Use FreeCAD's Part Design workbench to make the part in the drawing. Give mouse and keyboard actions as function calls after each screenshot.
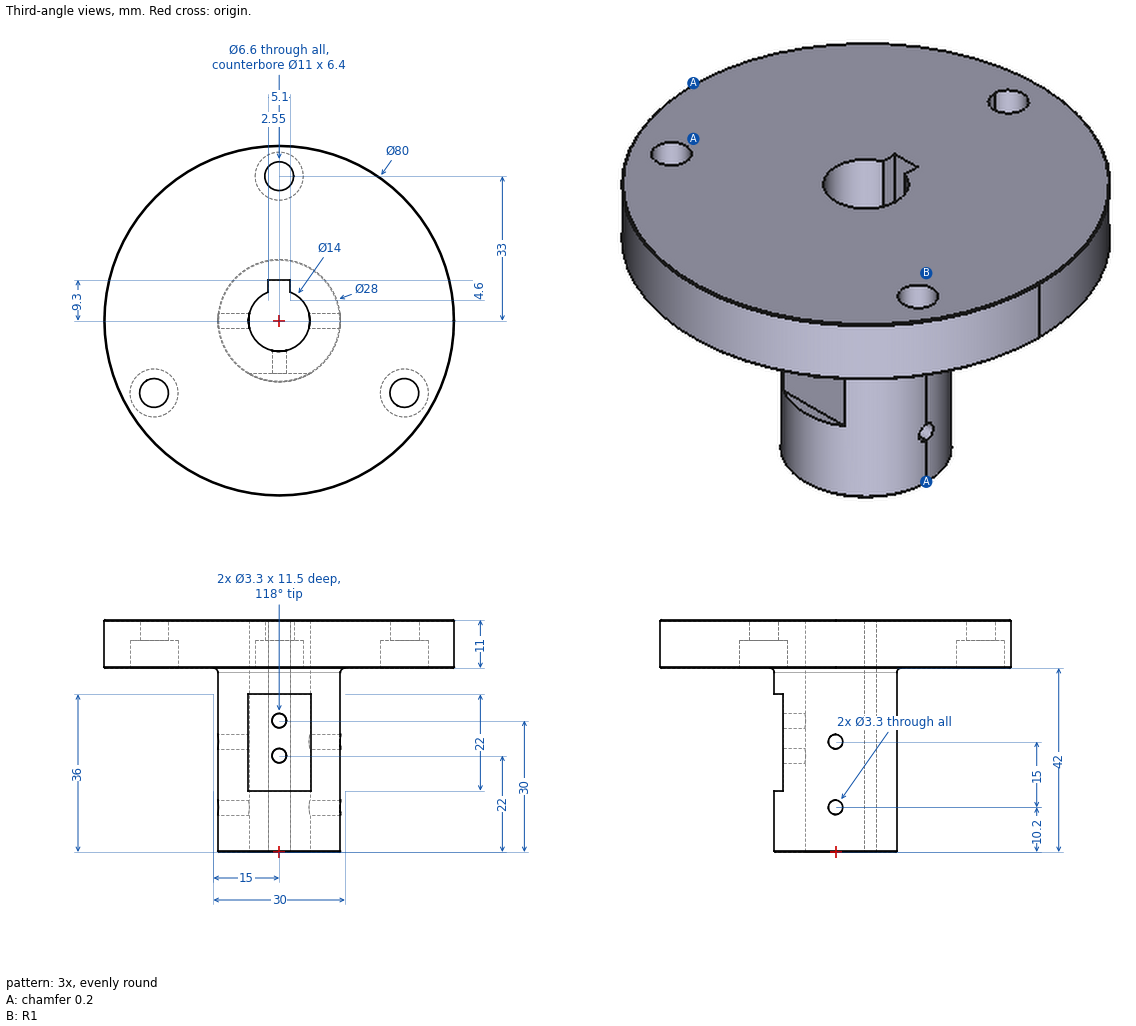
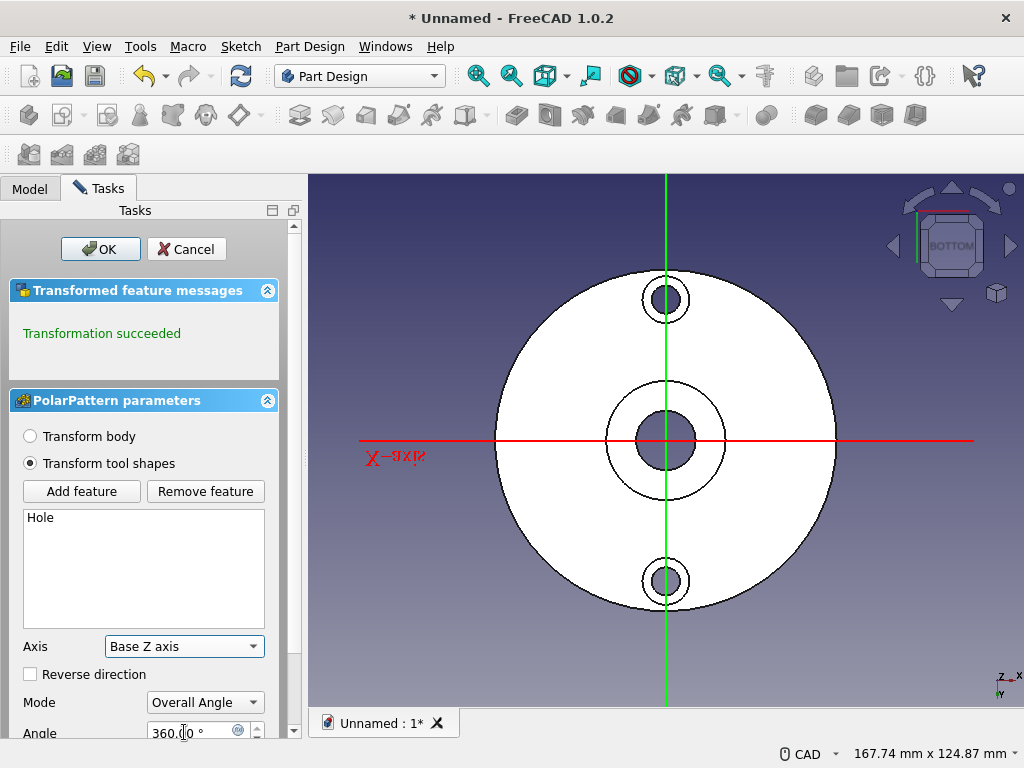
scroll(294, 479, down, 2)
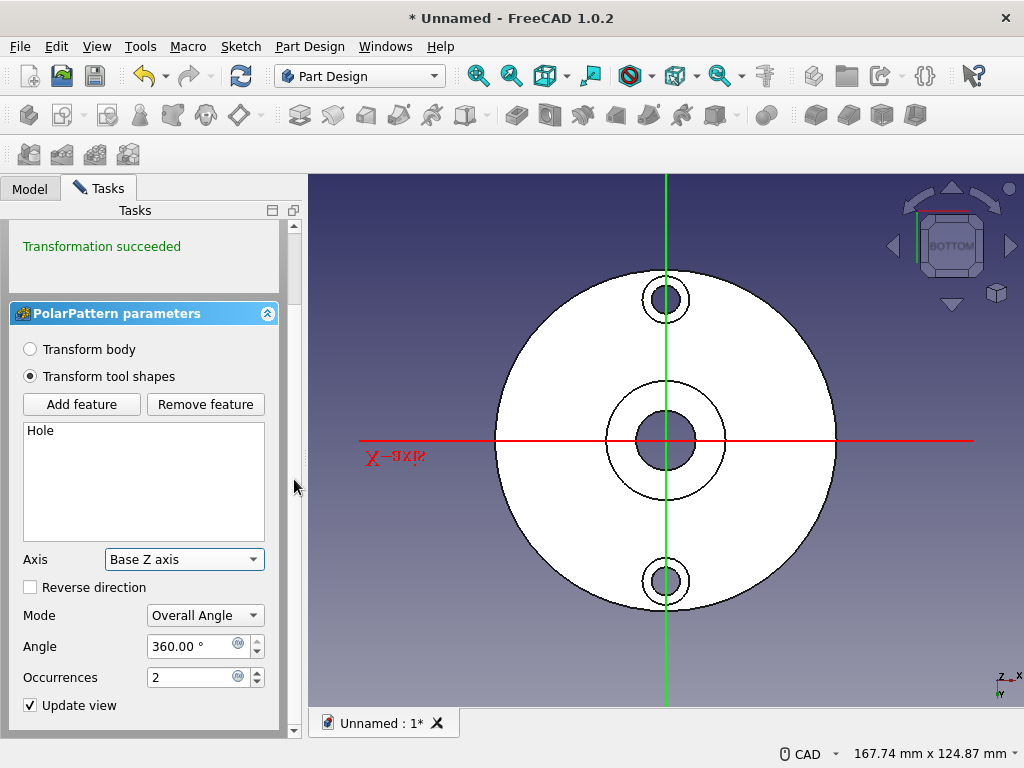
triple_click(199, 678)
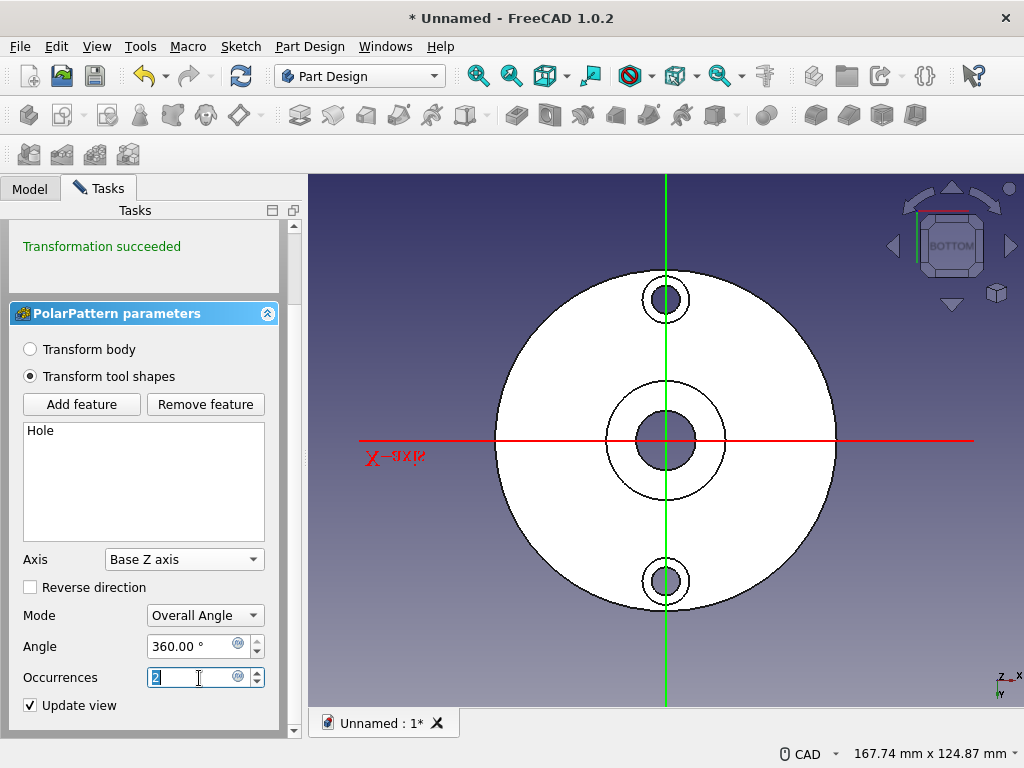
text(3)
key(Tab)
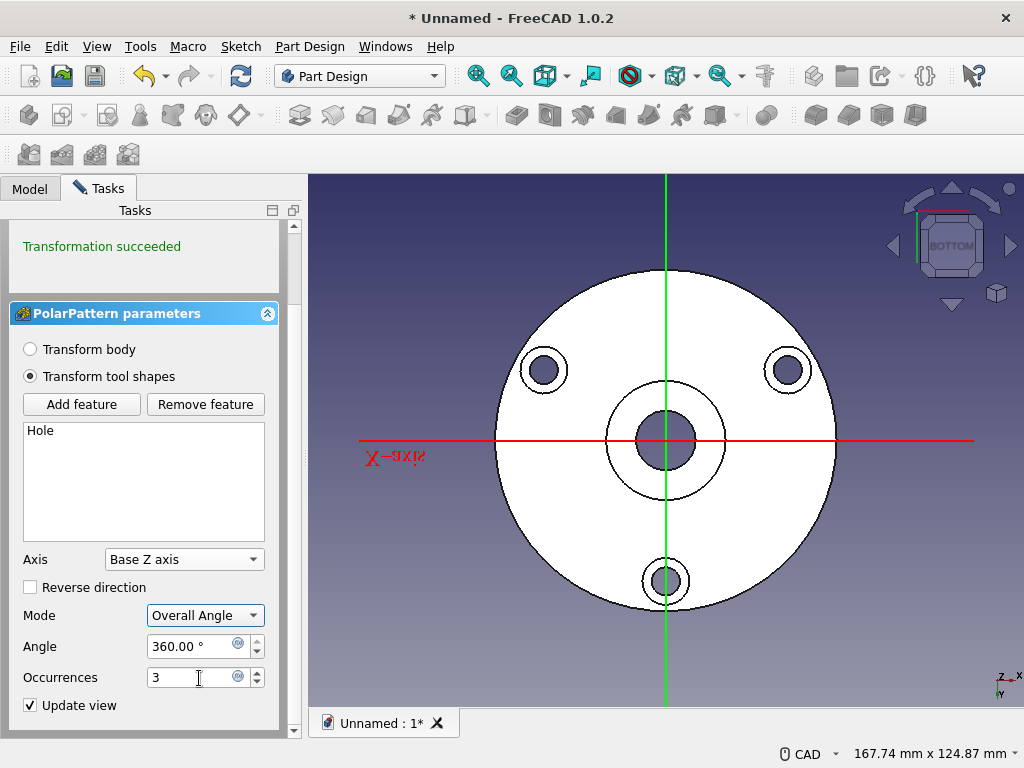
scroll(294, 479, up, 3)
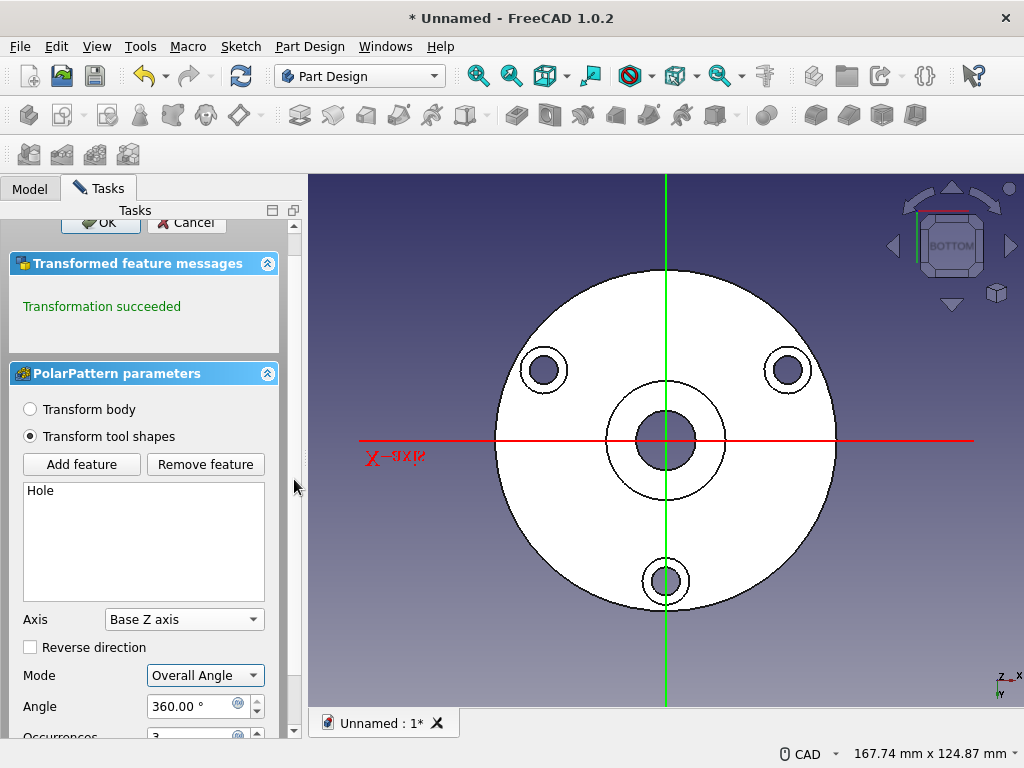
click(101, 249)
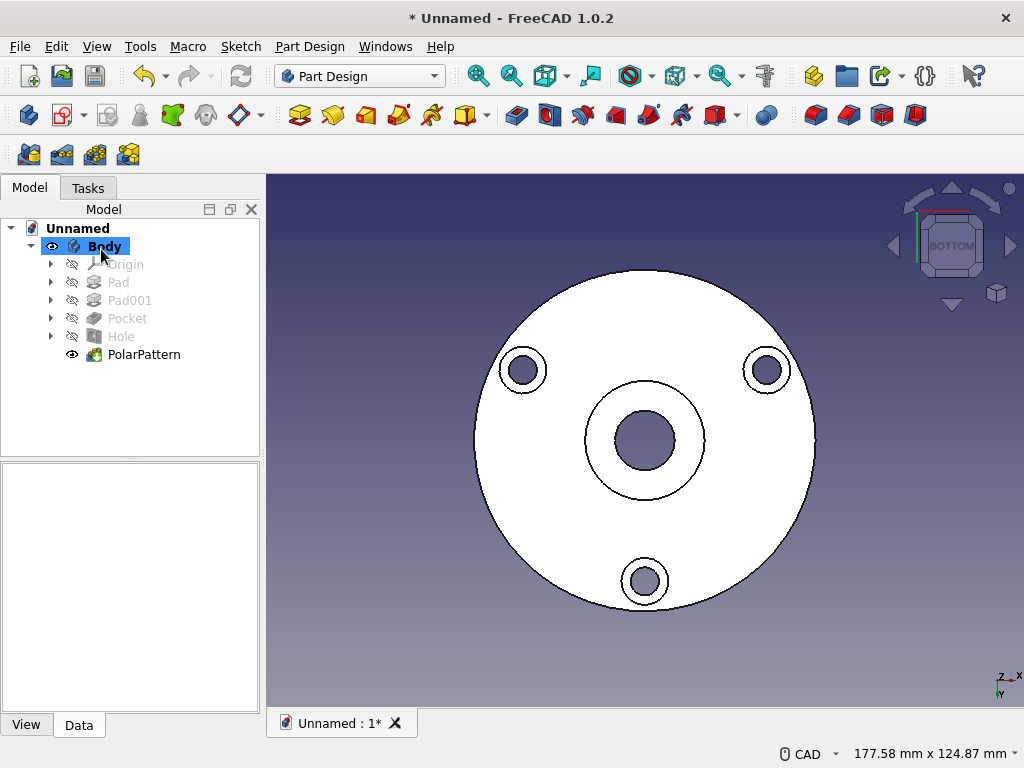
click(51, 264)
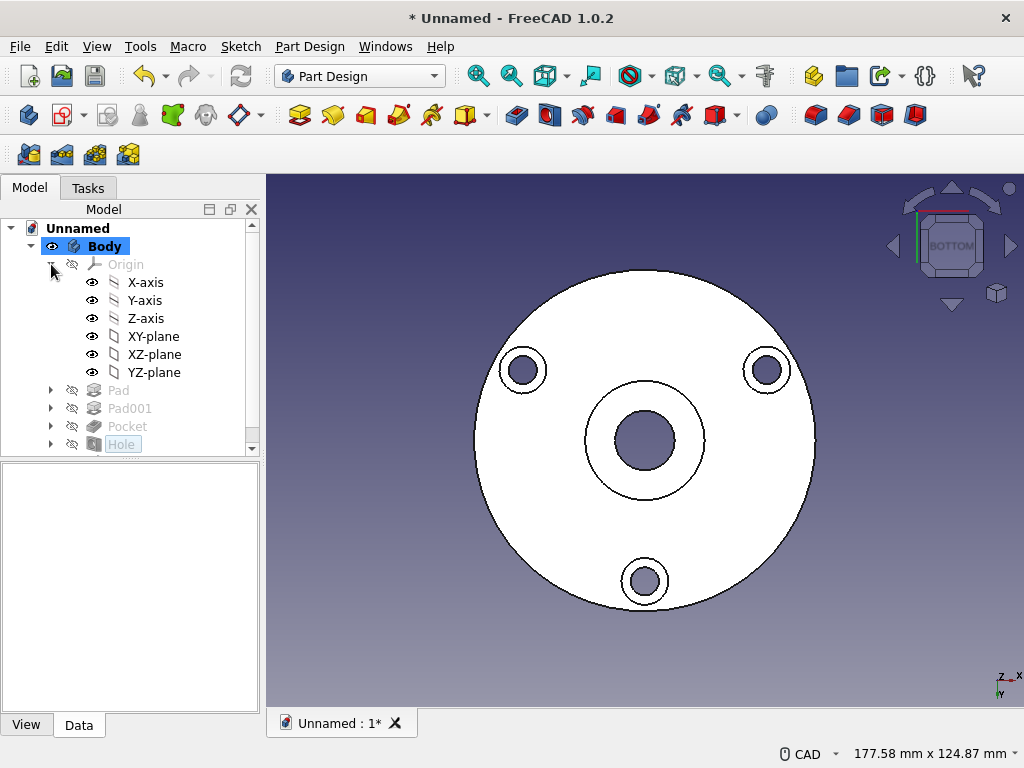
click(137, 354)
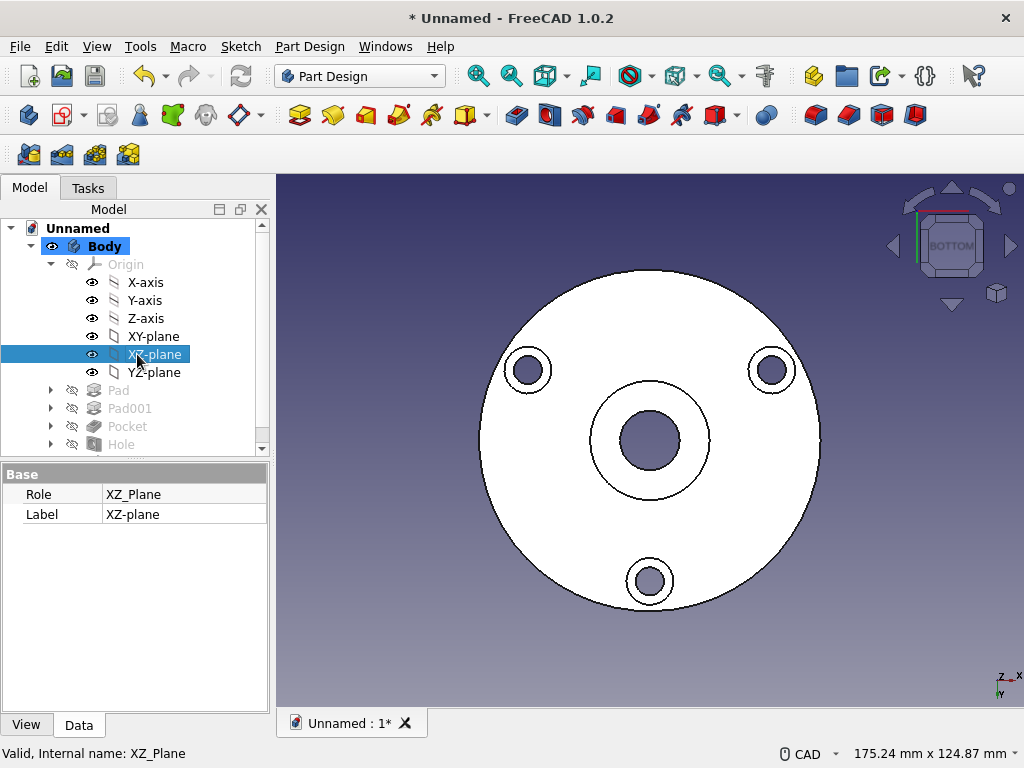
click(238, 116)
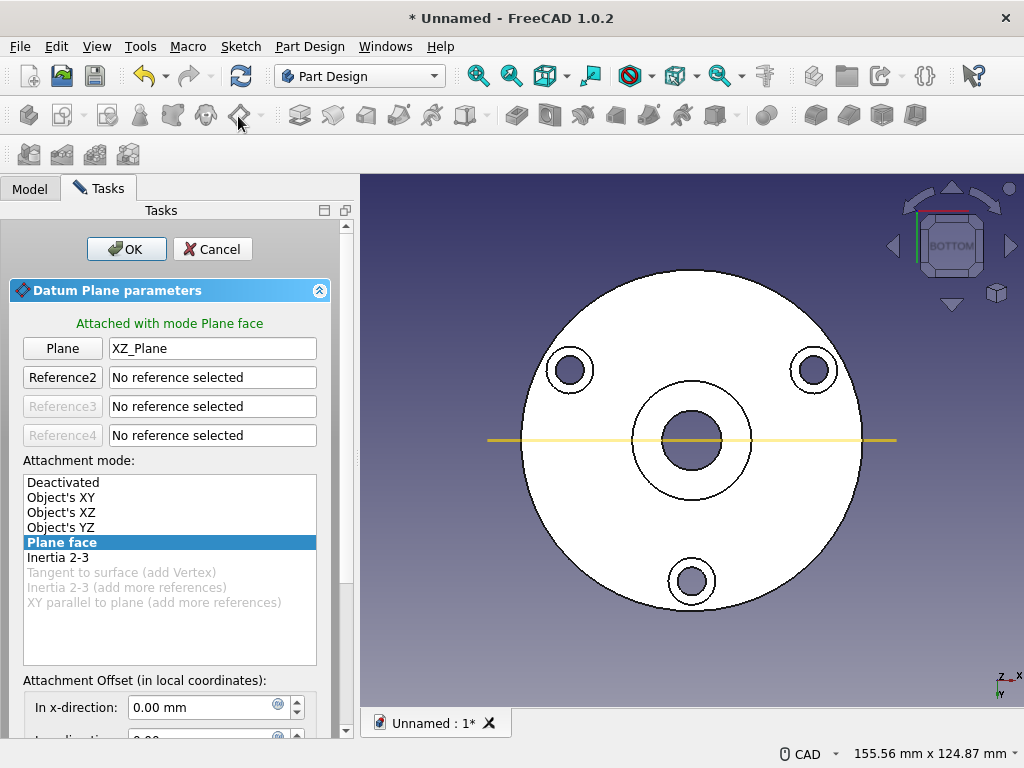
scroll(346, 479, down, 2)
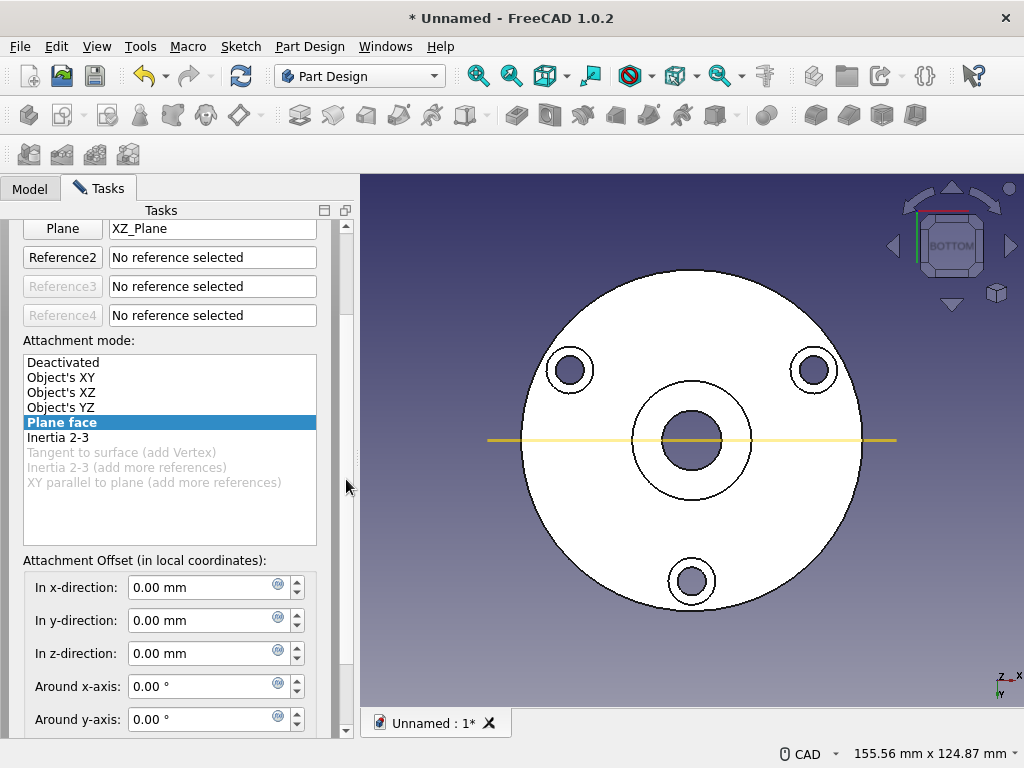
triple_click(210, 654)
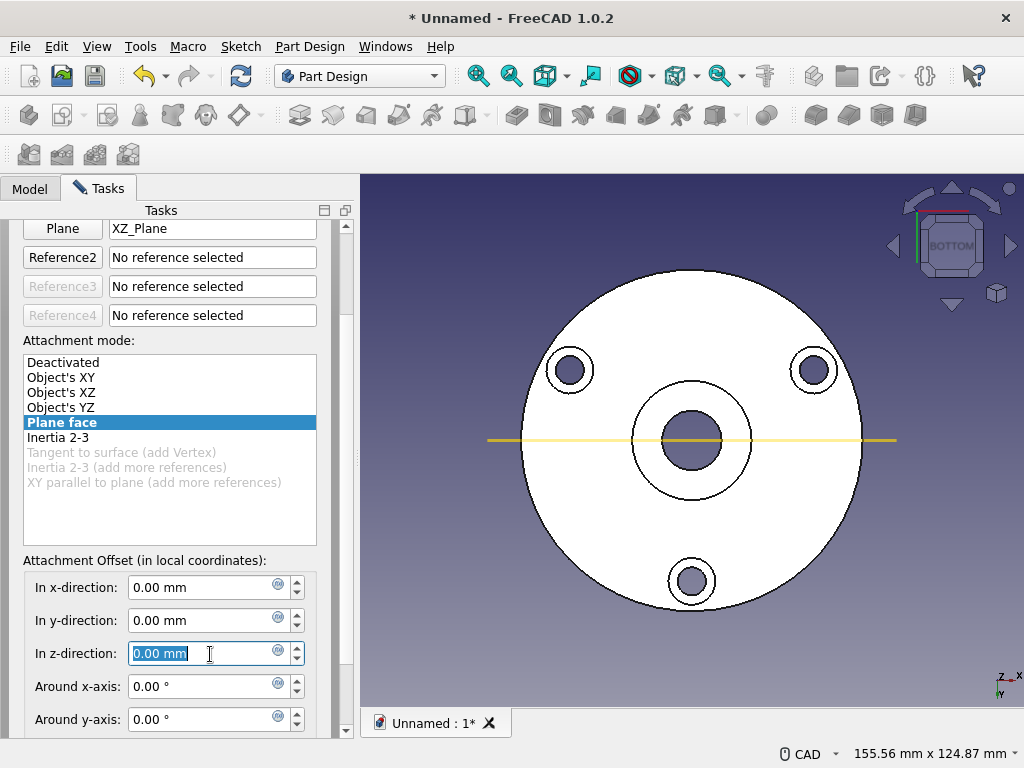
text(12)
key(Tab)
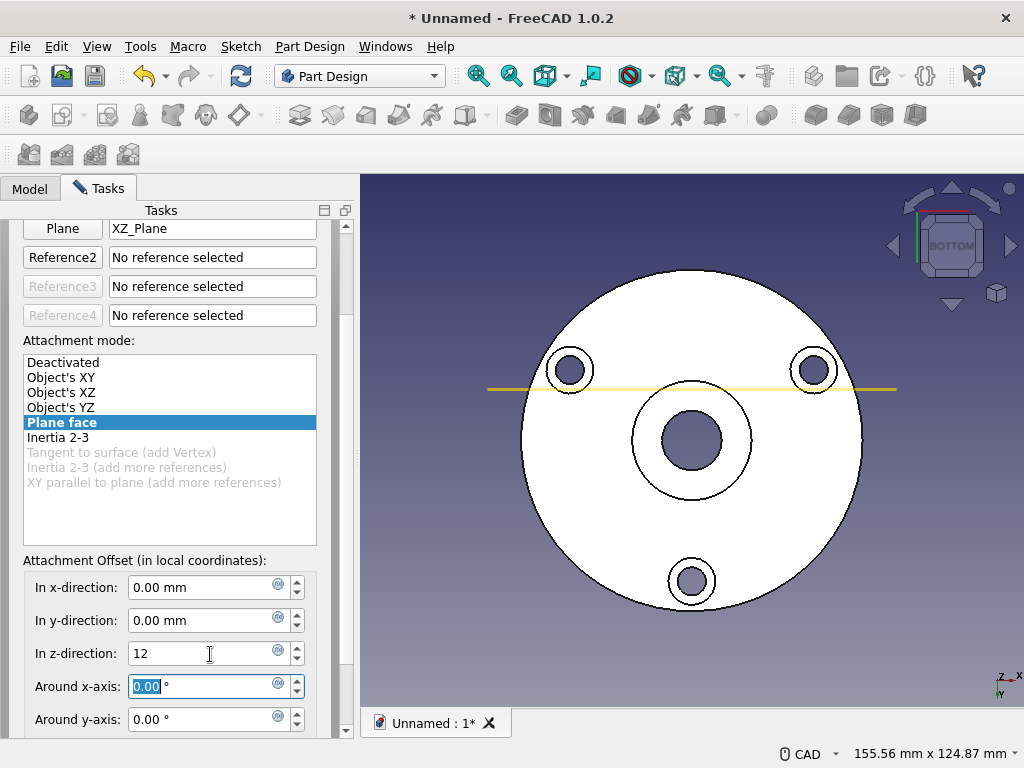
scroll(346, 479, up, 3)